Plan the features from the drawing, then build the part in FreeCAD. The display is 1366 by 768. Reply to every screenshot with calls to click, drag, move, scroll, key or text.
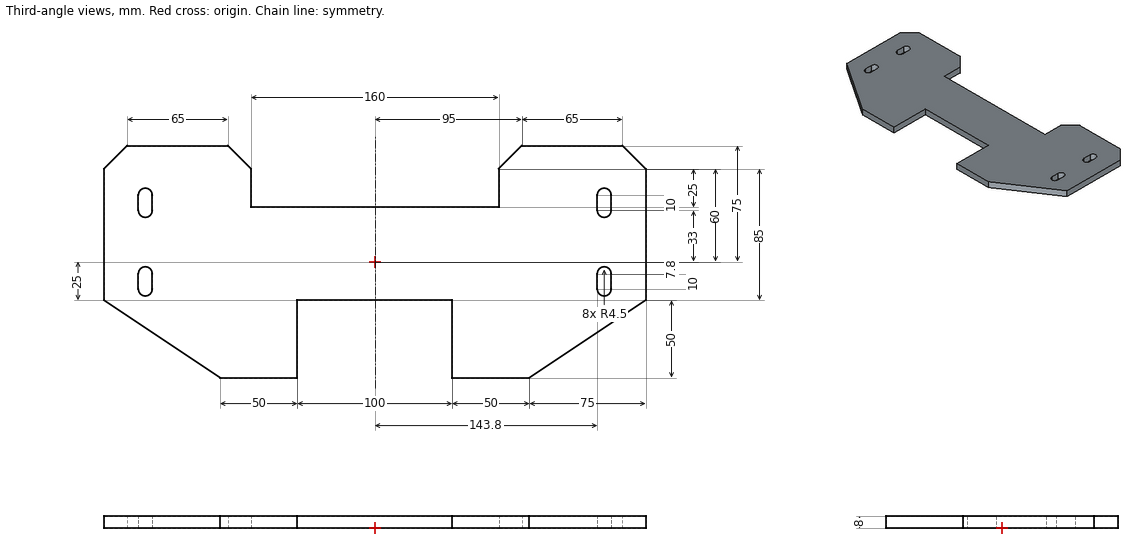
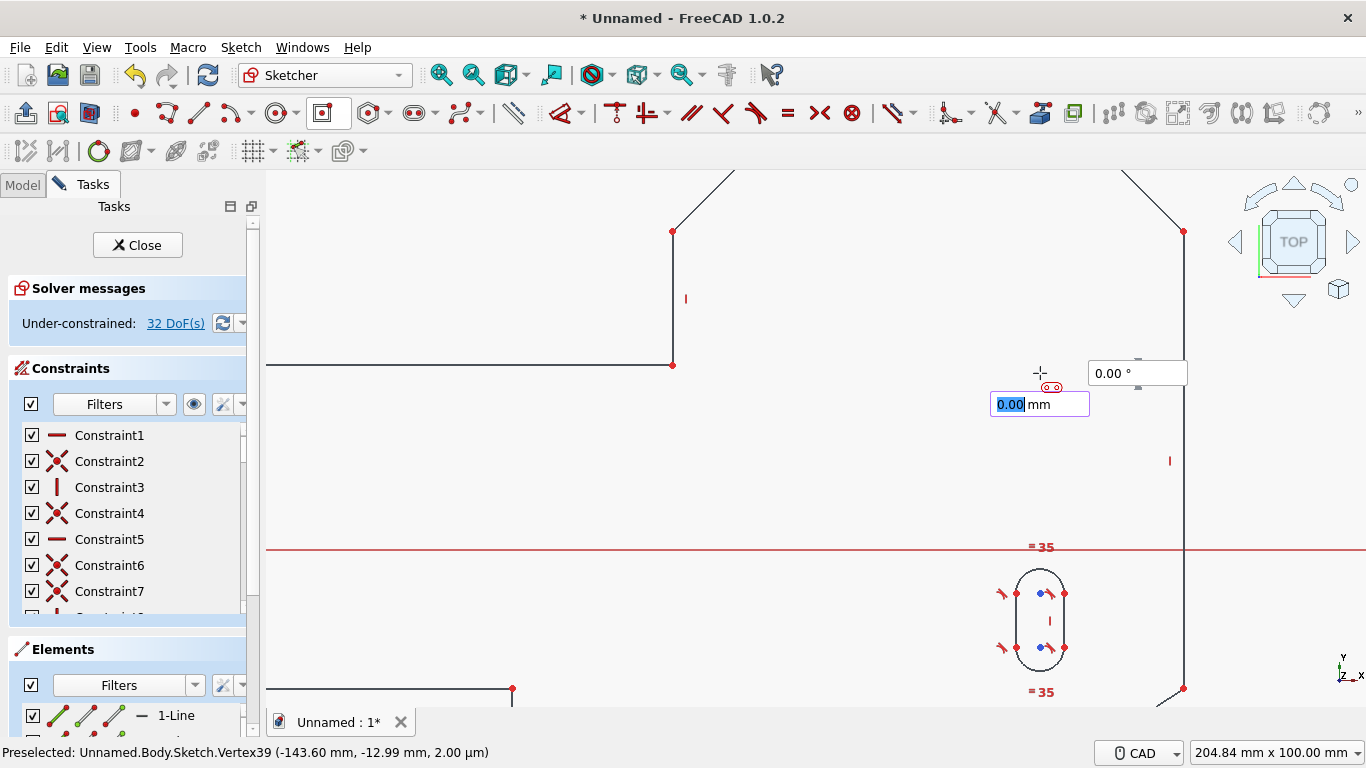
click(1040, 319)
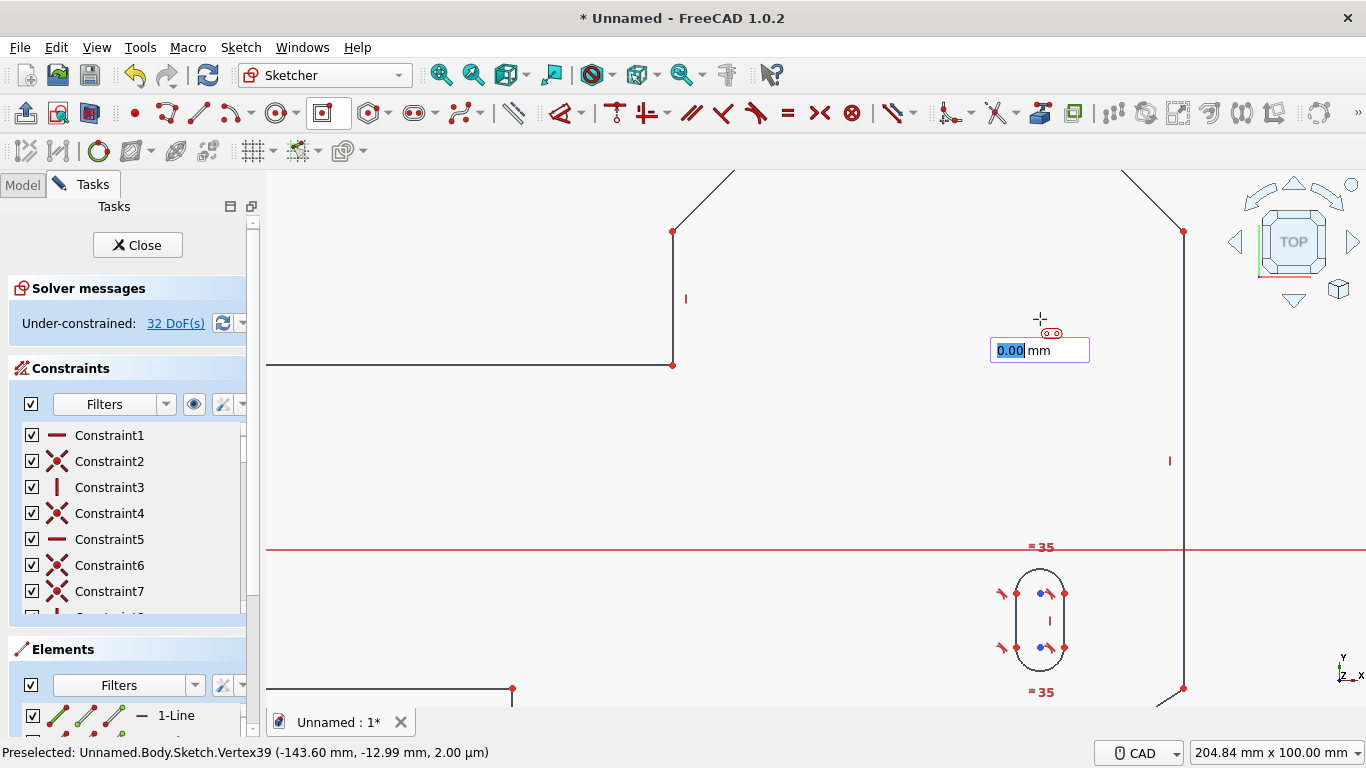
click(1064, 346)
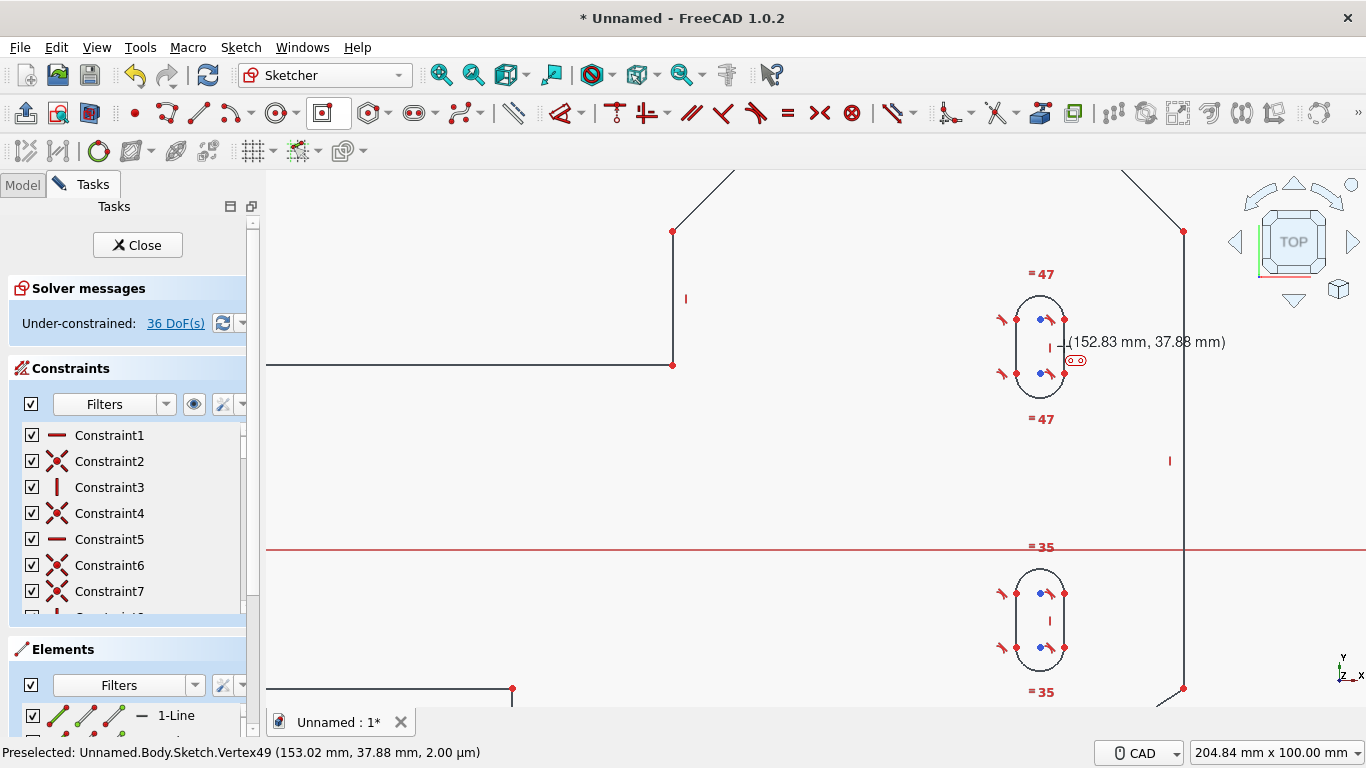
scroll(1041, 373, down, 5)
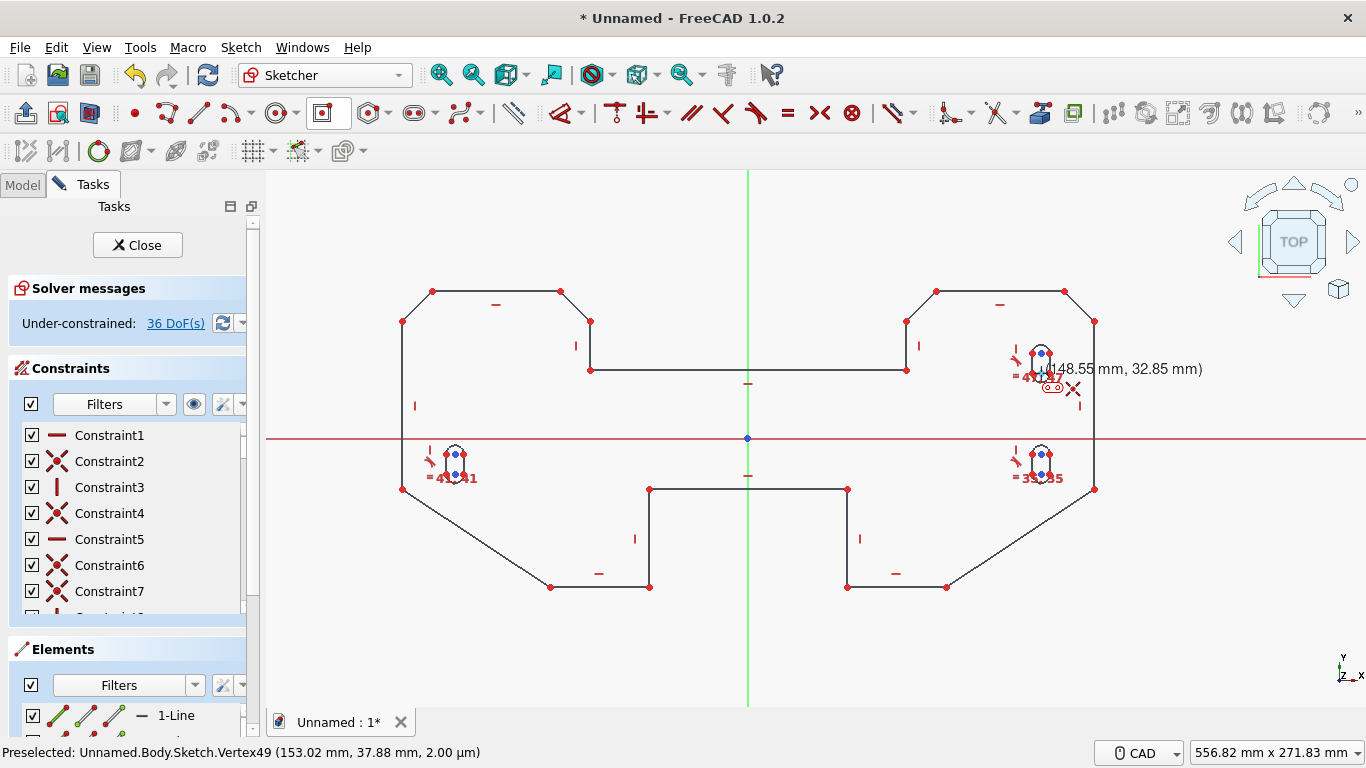
scroll(455, 373, up, 5)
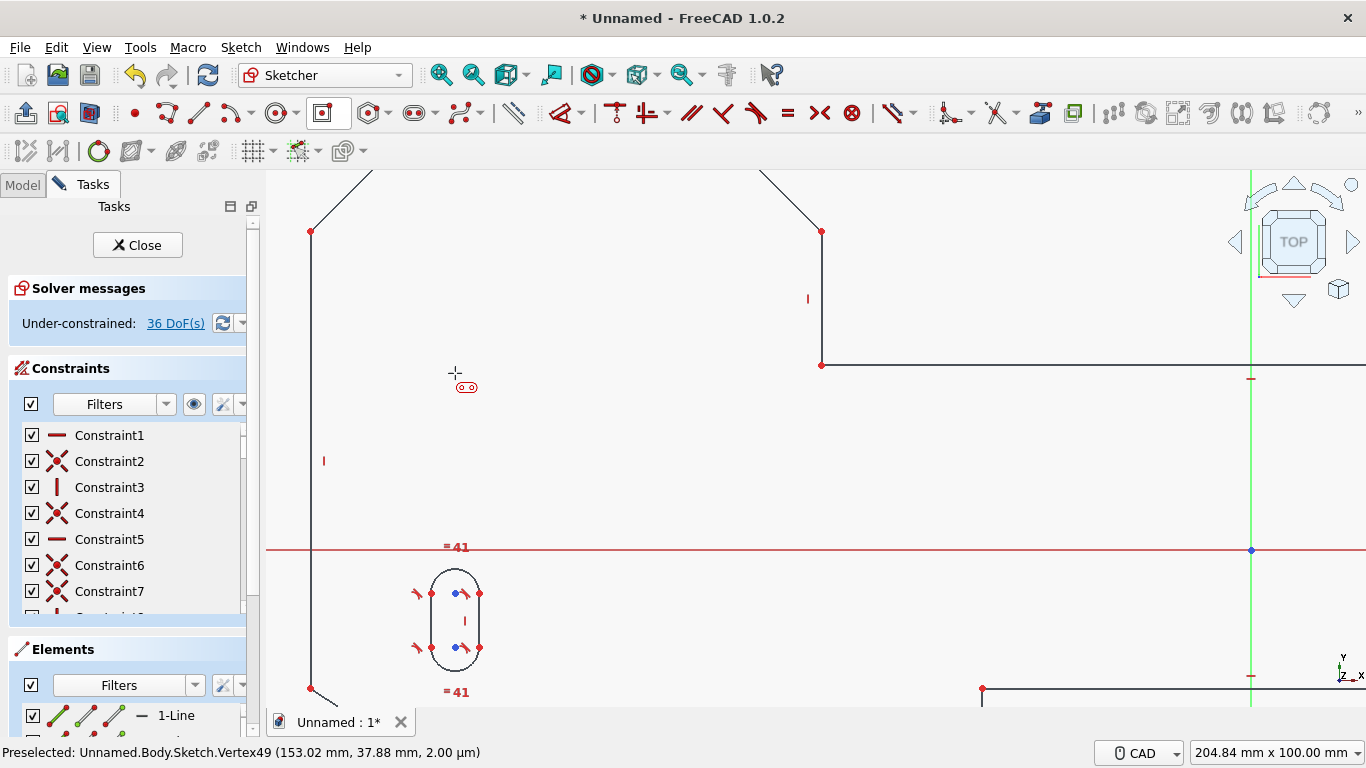
click(455, 373)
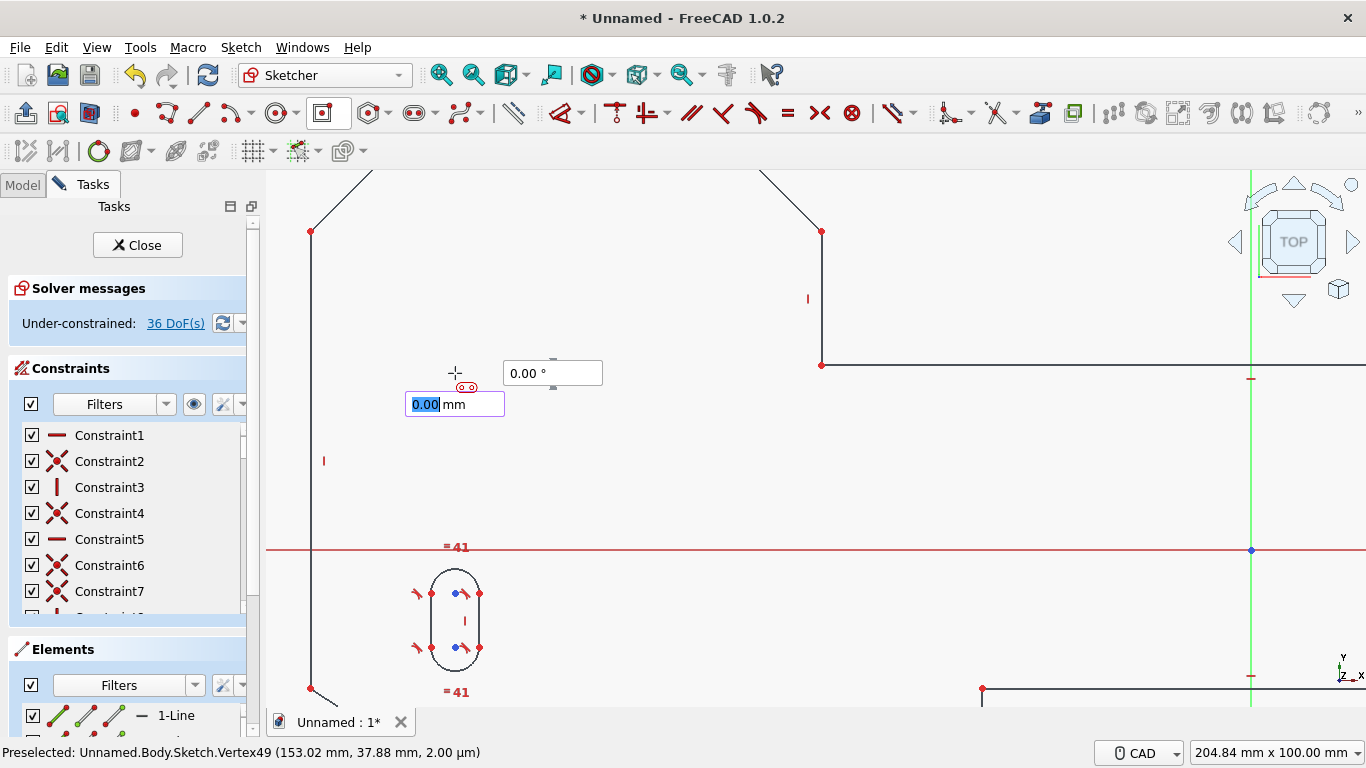
click(455, 319)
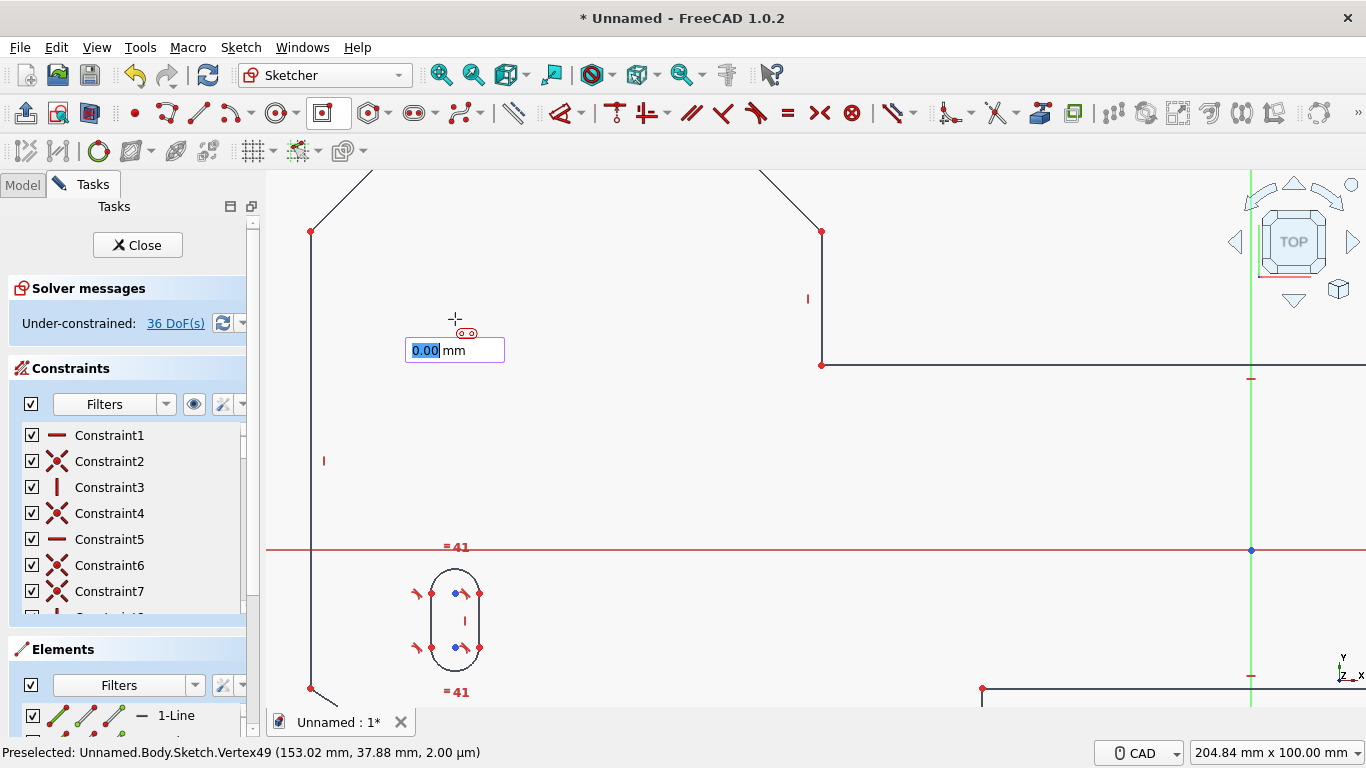
click(479, 346)
key(Escape)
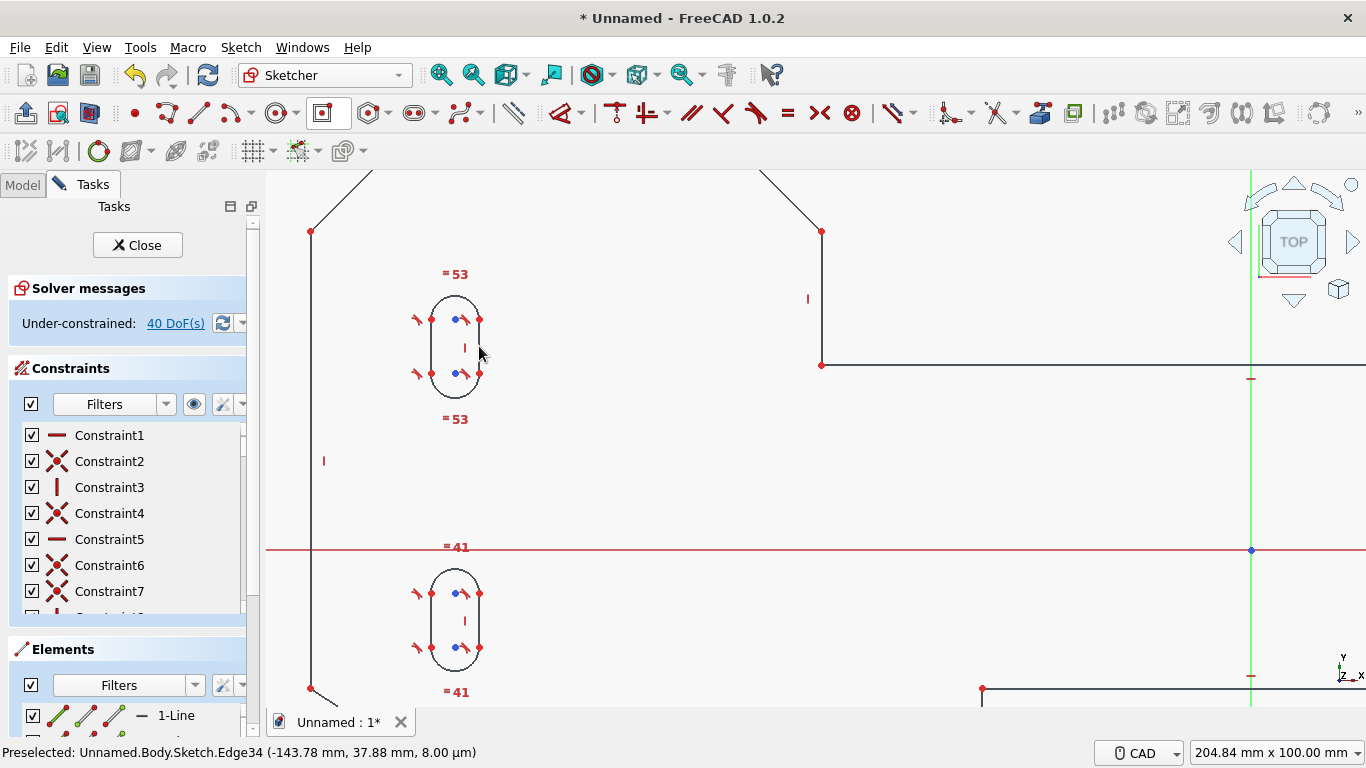
scroll(454, 373, down, 5)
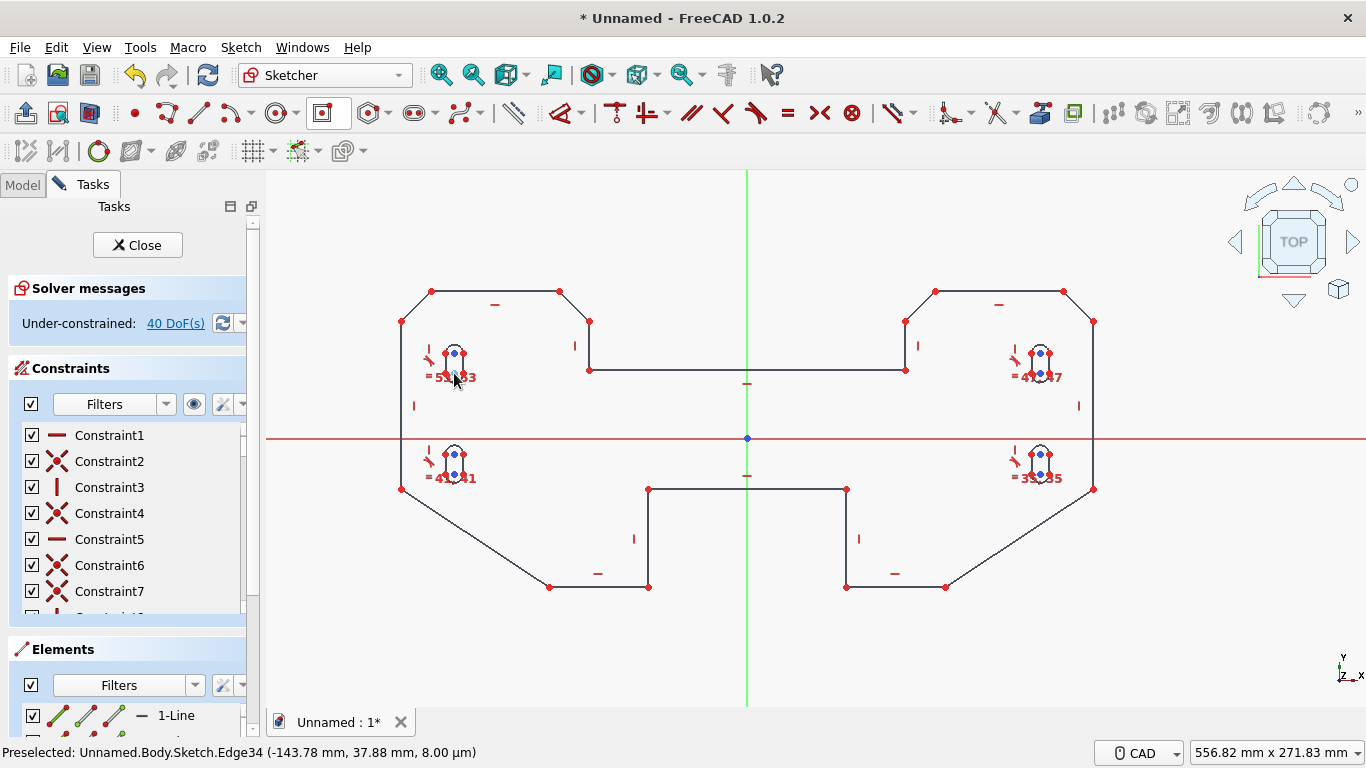
scroll(1035, 481, up, 3)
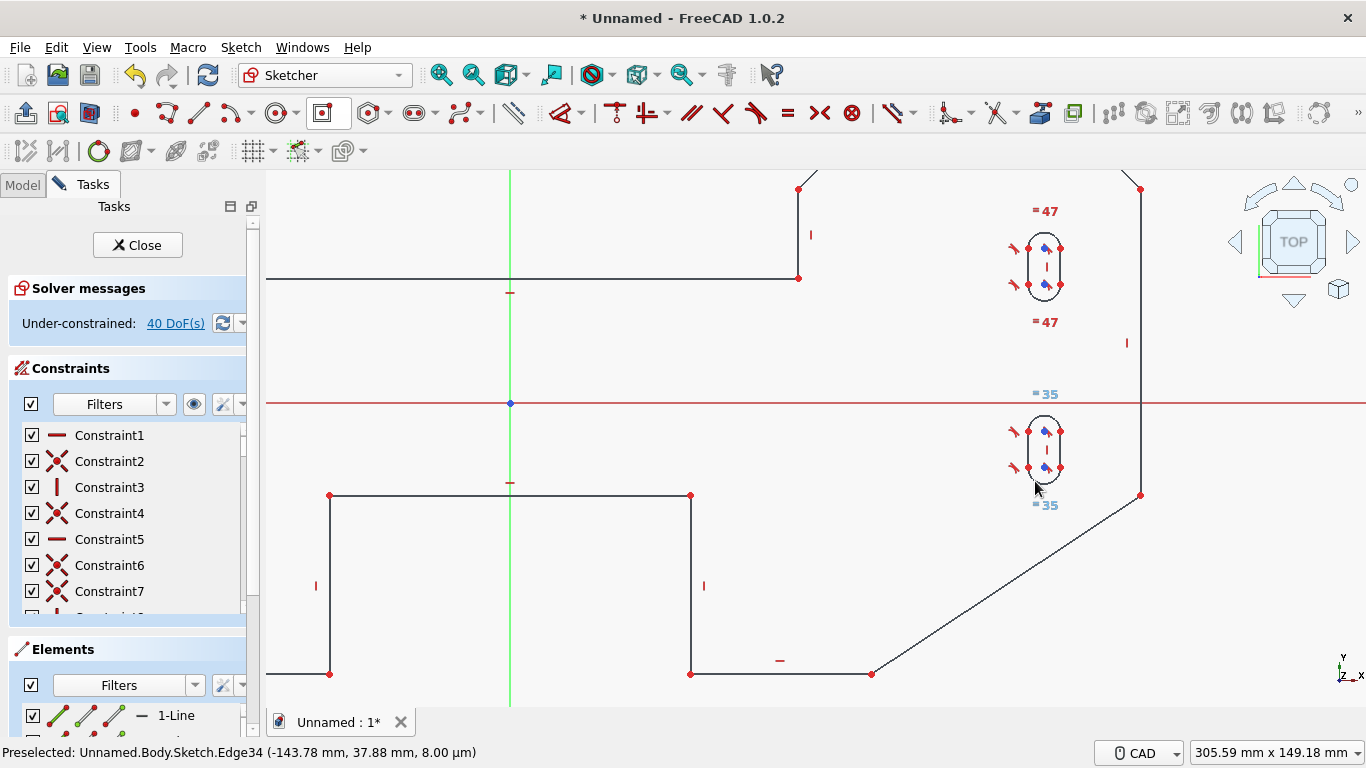
click(1035, 481)